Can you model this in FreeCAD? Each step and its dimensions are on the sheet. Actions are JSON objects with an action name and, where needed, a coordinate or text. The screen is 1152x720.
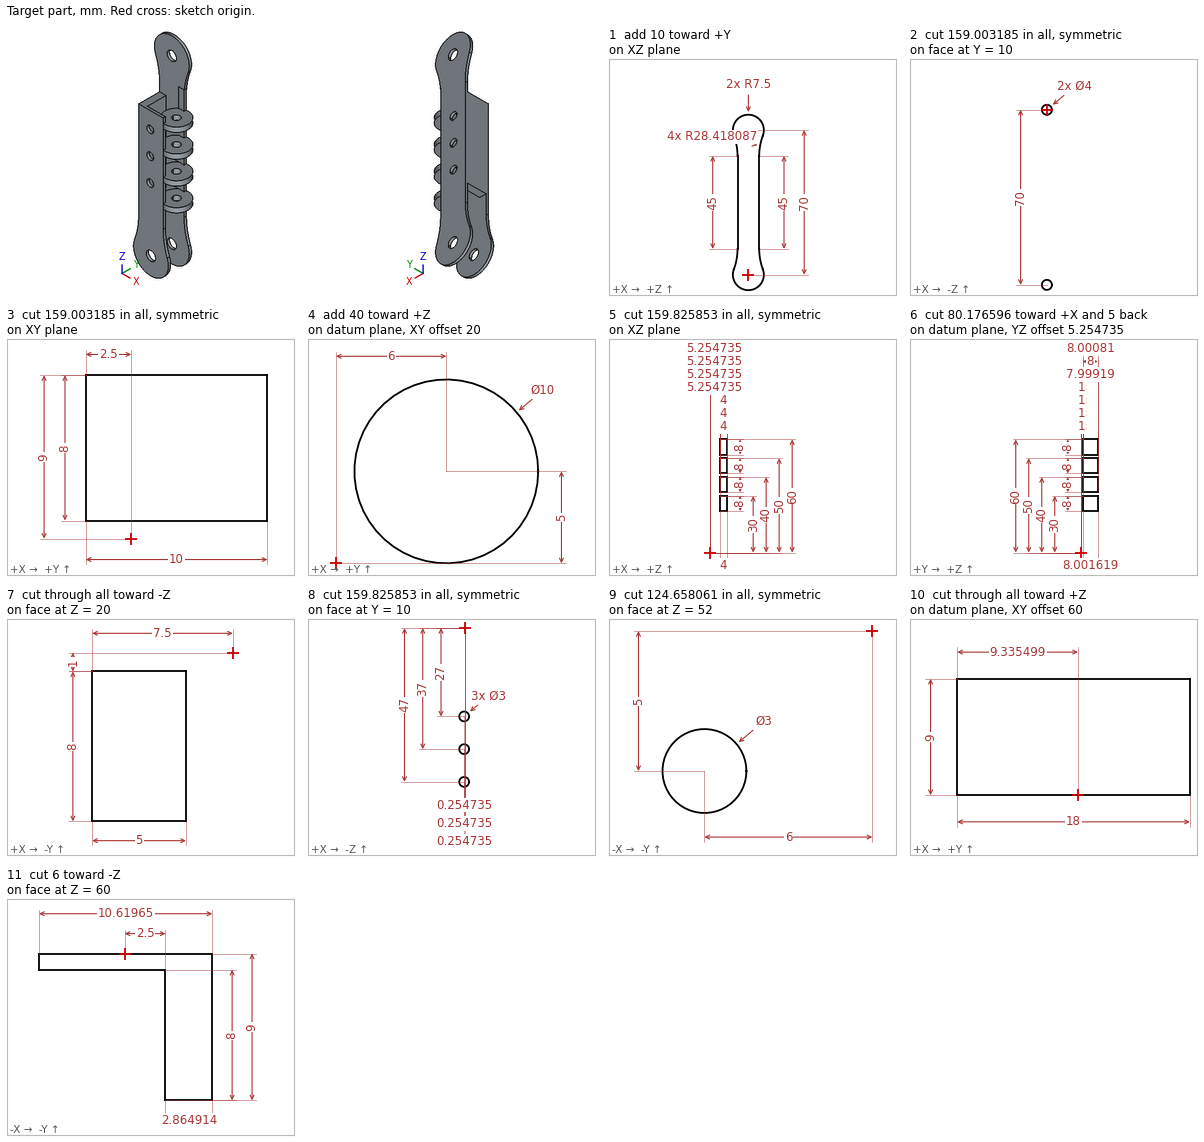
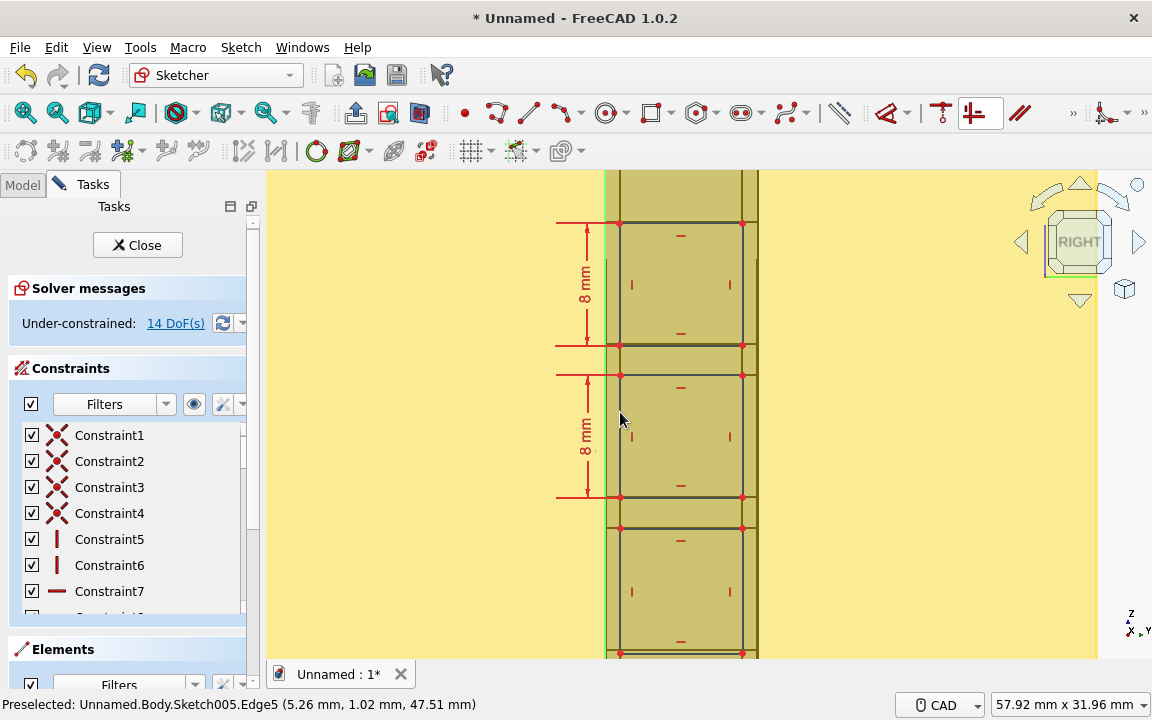
{"action": "left_click", "coordinate": [657, 498]}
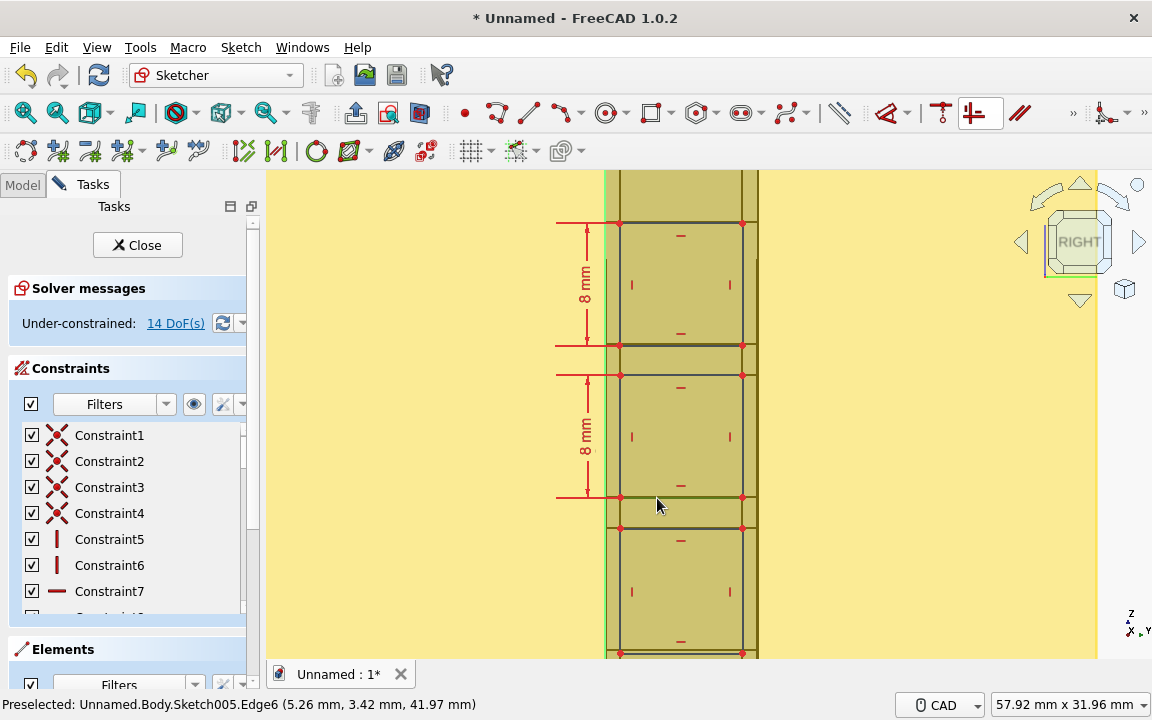
{"action": "left_click", "coordinate": [910, 114]}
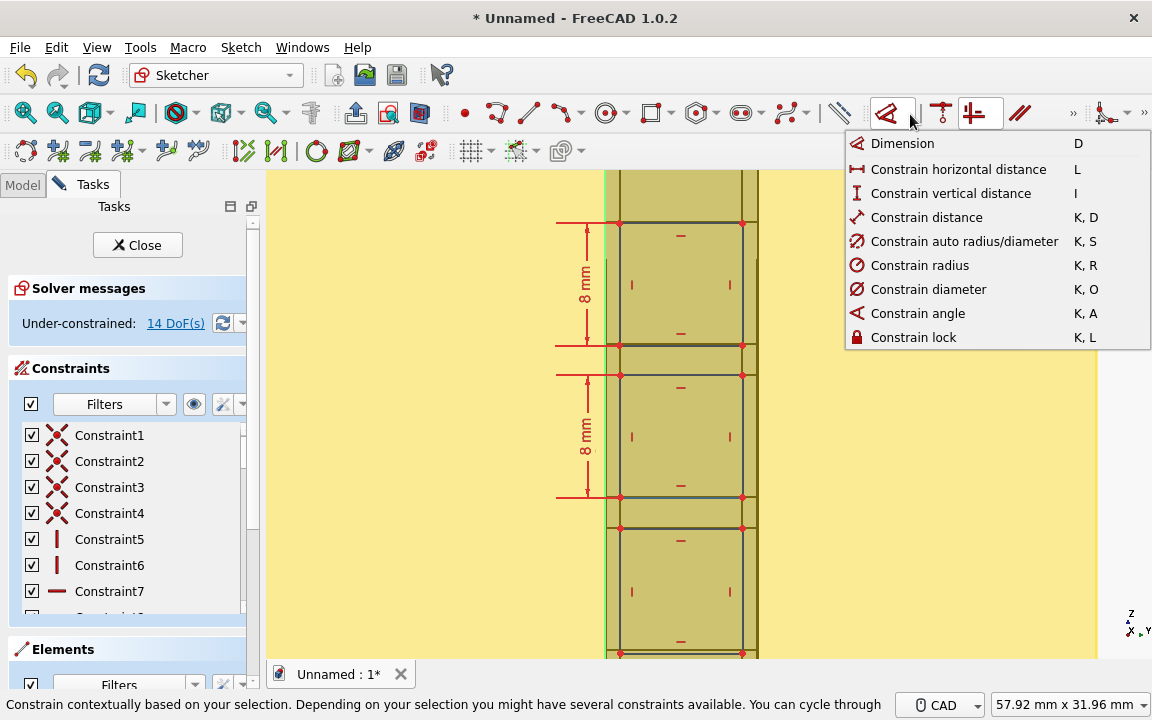
{"action": "left_click", "coordinate": [998, 169]}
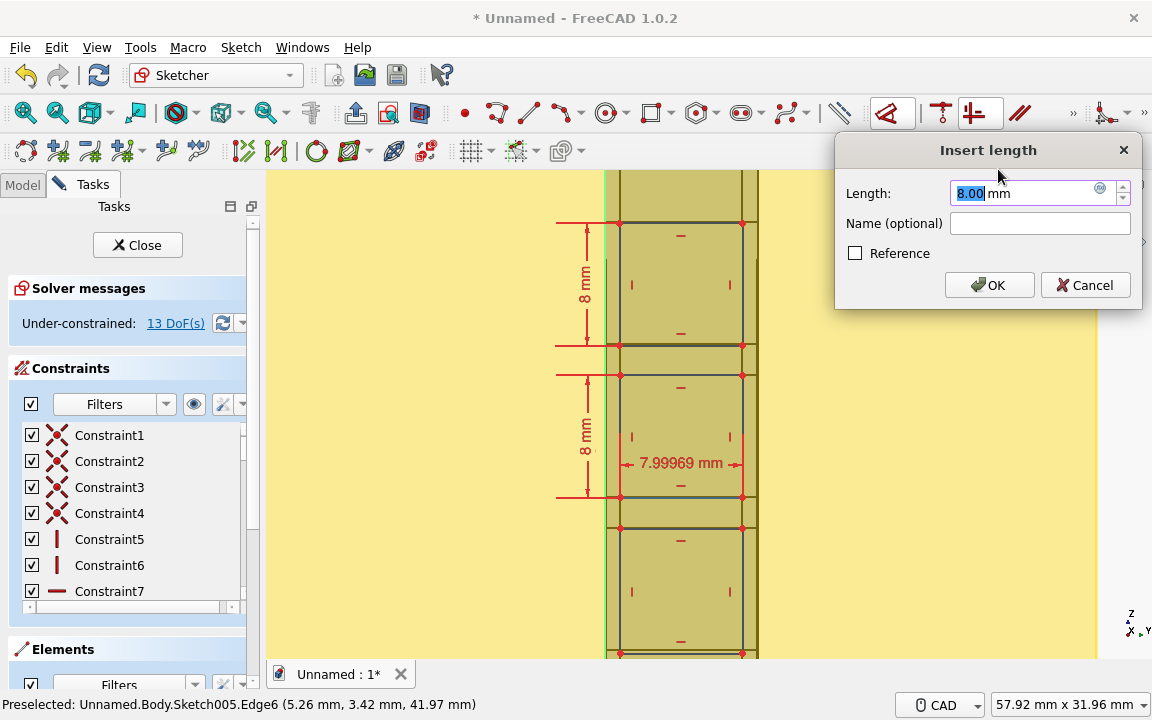
{"action": "type", "text": "8"}
{"action": "key", "text": "Return"}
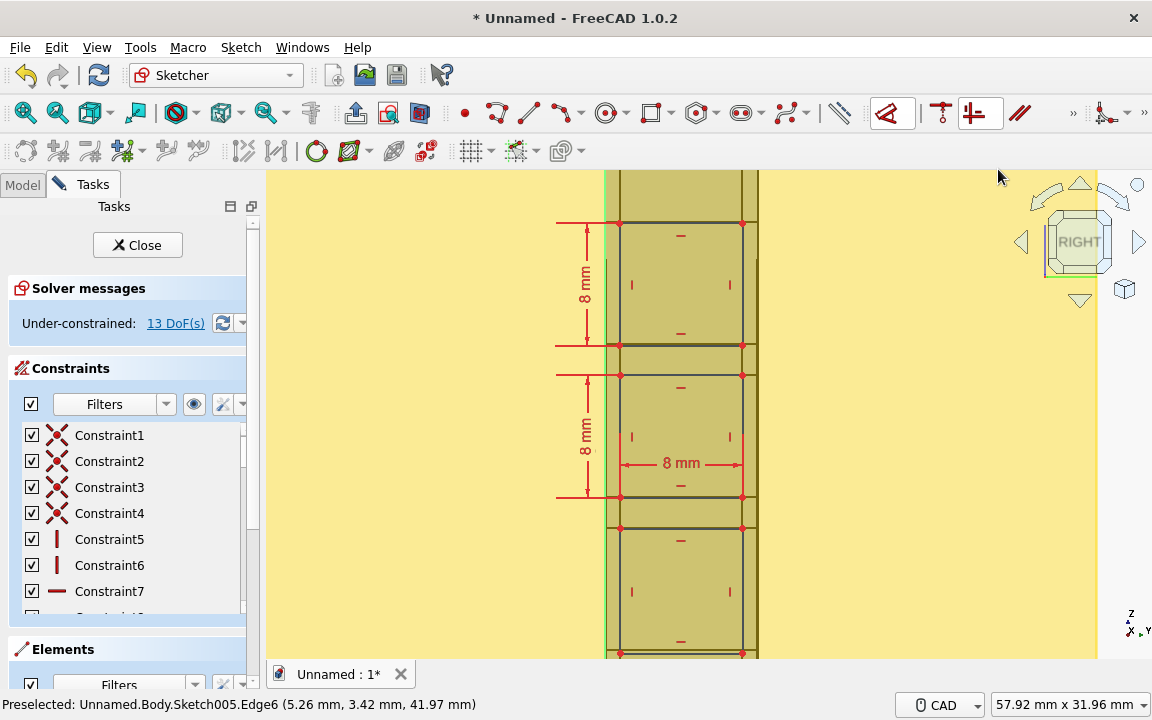
{"action": "left_click", "coordinate": [620, 566]}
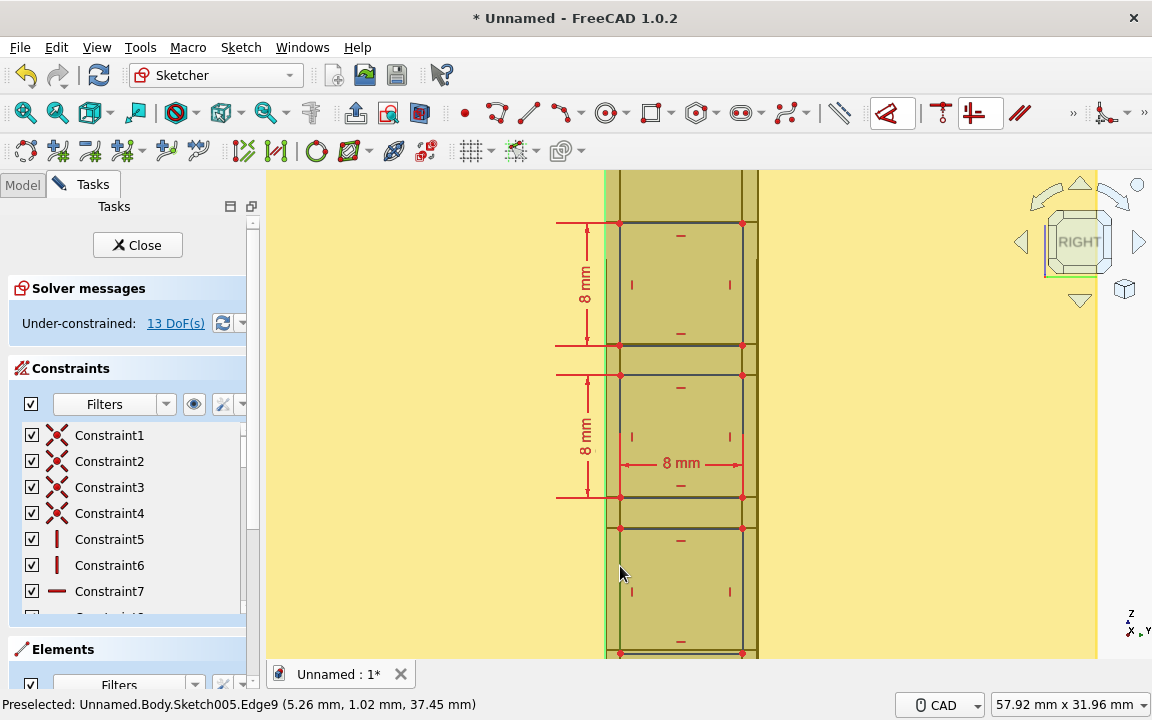
{"action": "left_click", "coordinate": [910, 114]}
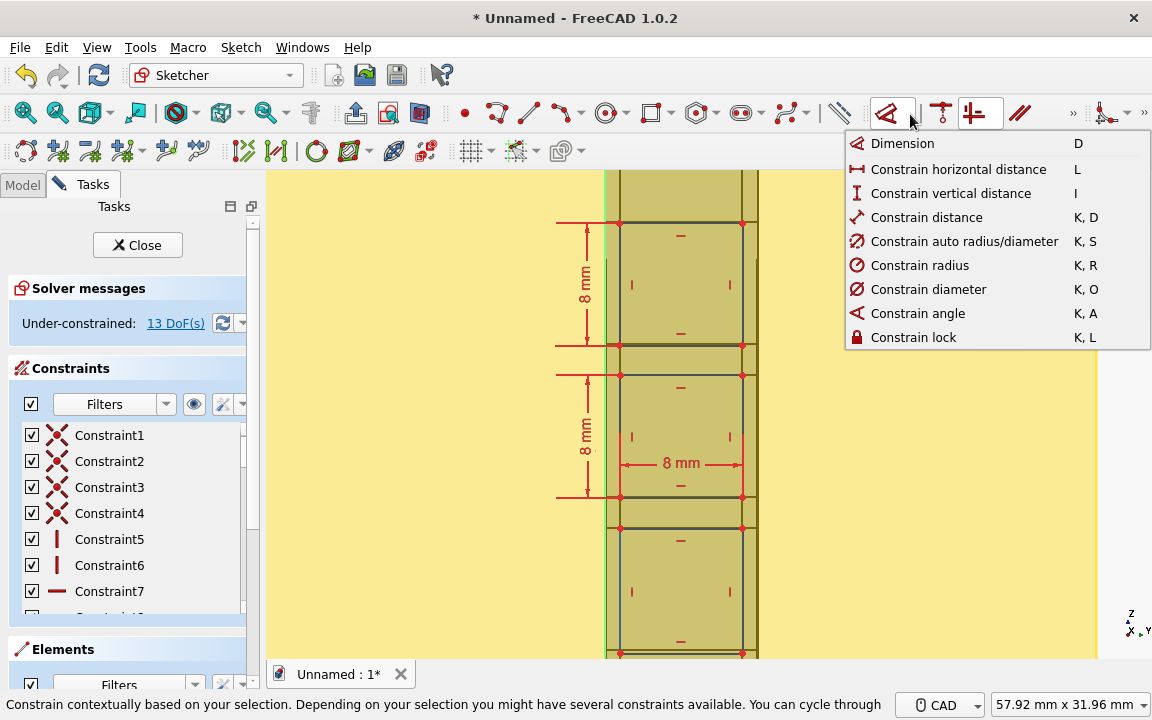
{"action": "left_click", "coordinate": [998, 193]}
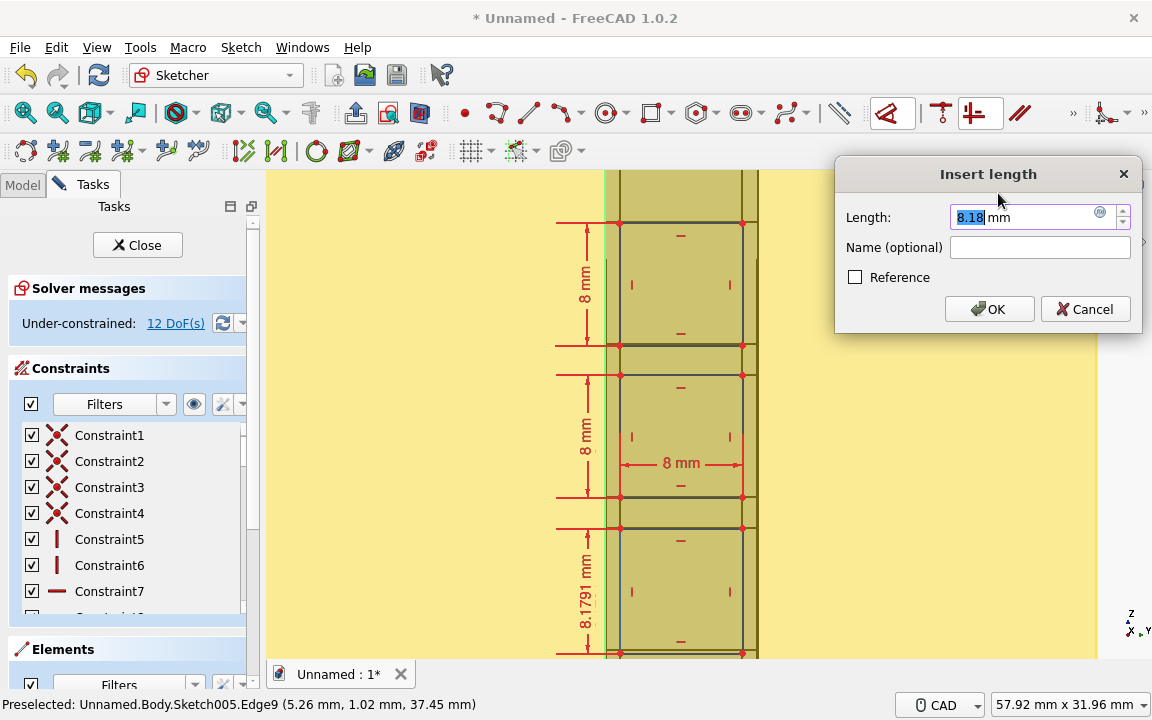
{"action": "type", "text": "8"}
{"action": "key", "text": "Return"}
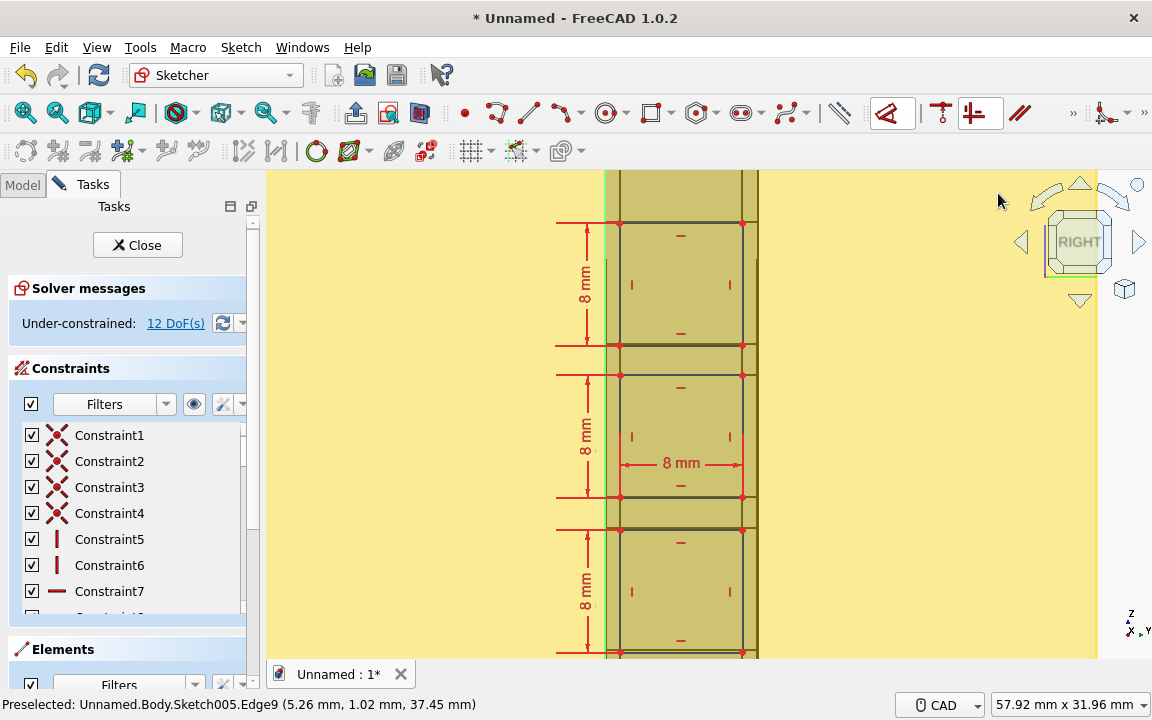
{"action": "scroll", "coordinate": [621, 259], "scroll_direction": "down", "scroll_amount": 5}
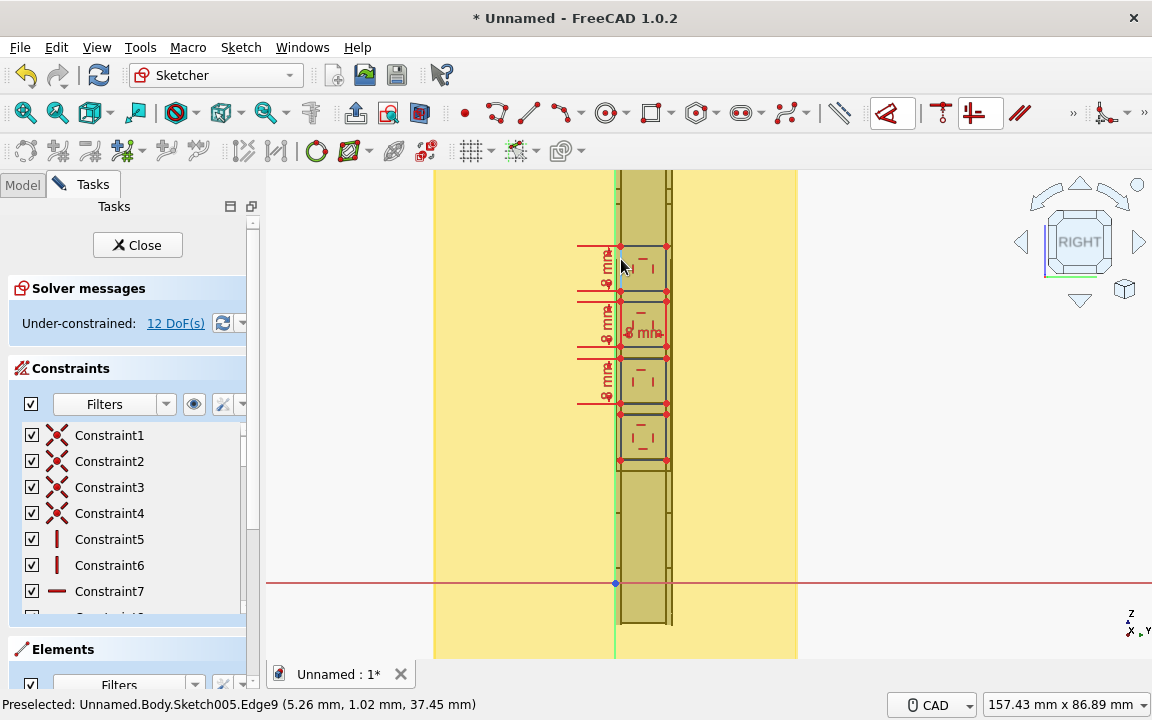
{"action": "scroll", "coordinate": [621, 428], "scroll_direction": "up", "scroll_amount": 5}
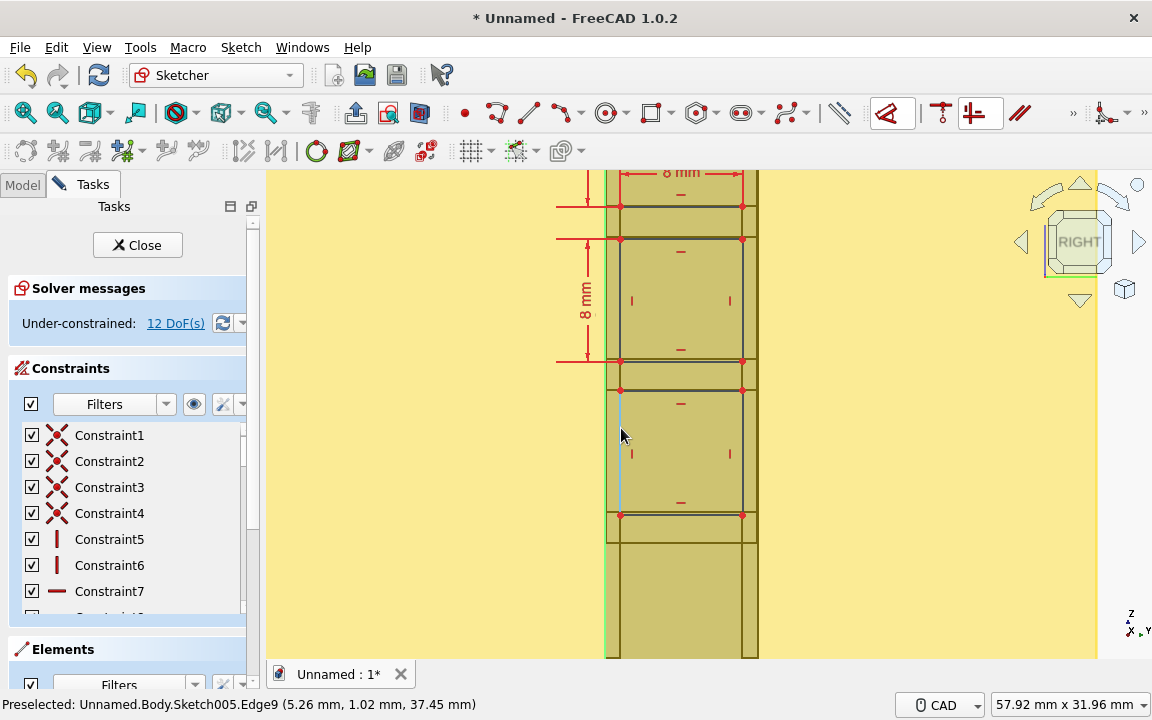
{"action": "left_click", "coordinate": [620, 428]}